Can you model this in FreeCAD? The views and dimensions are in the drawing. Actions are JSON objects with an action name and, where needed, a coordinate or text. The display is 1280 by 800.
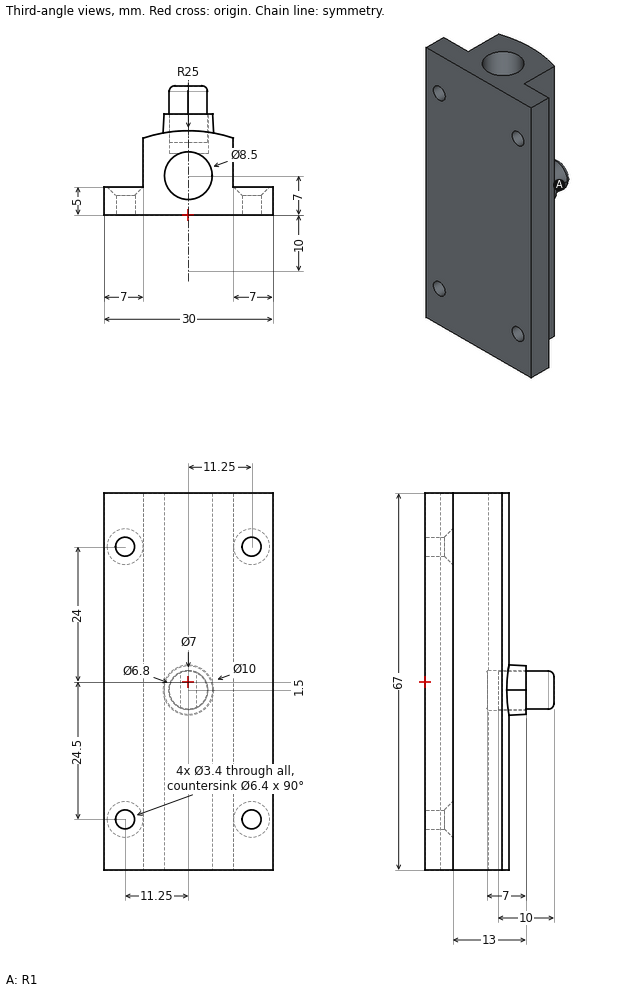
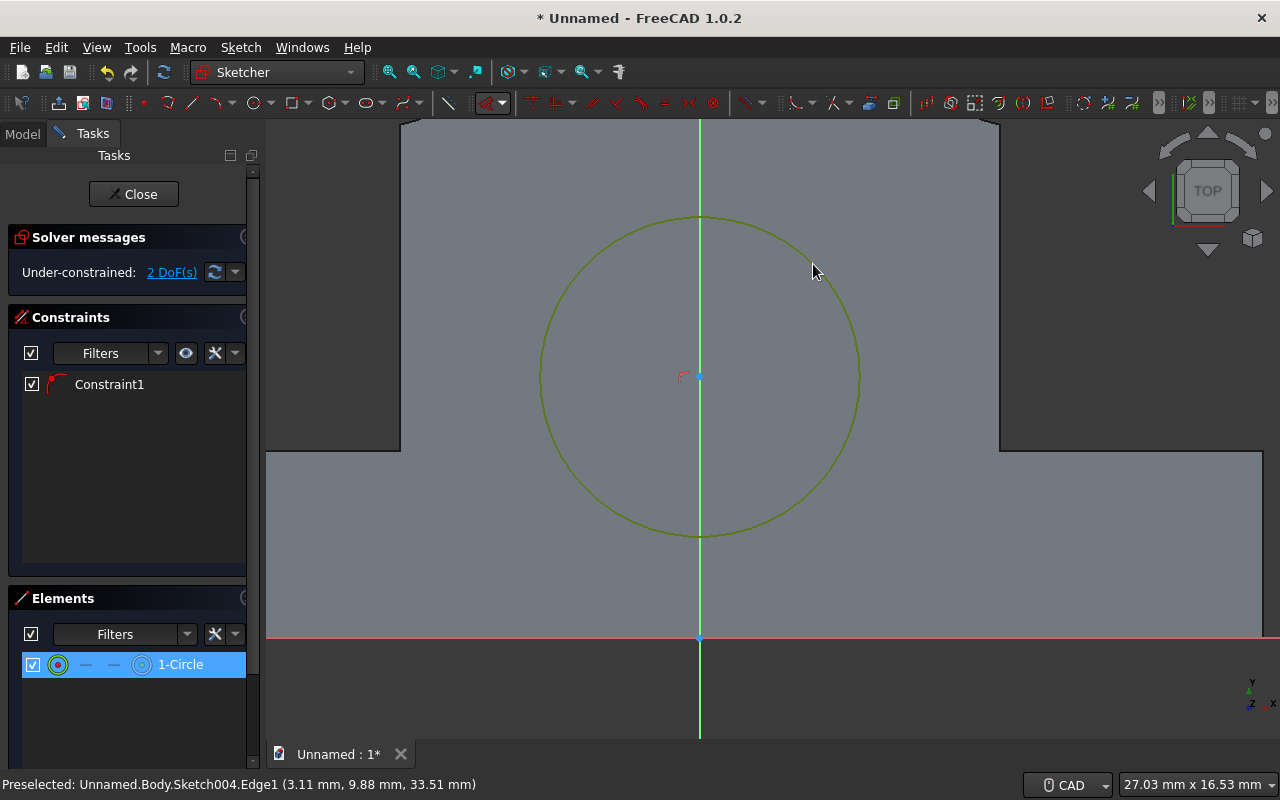
{"action": "key", "text": "k o"}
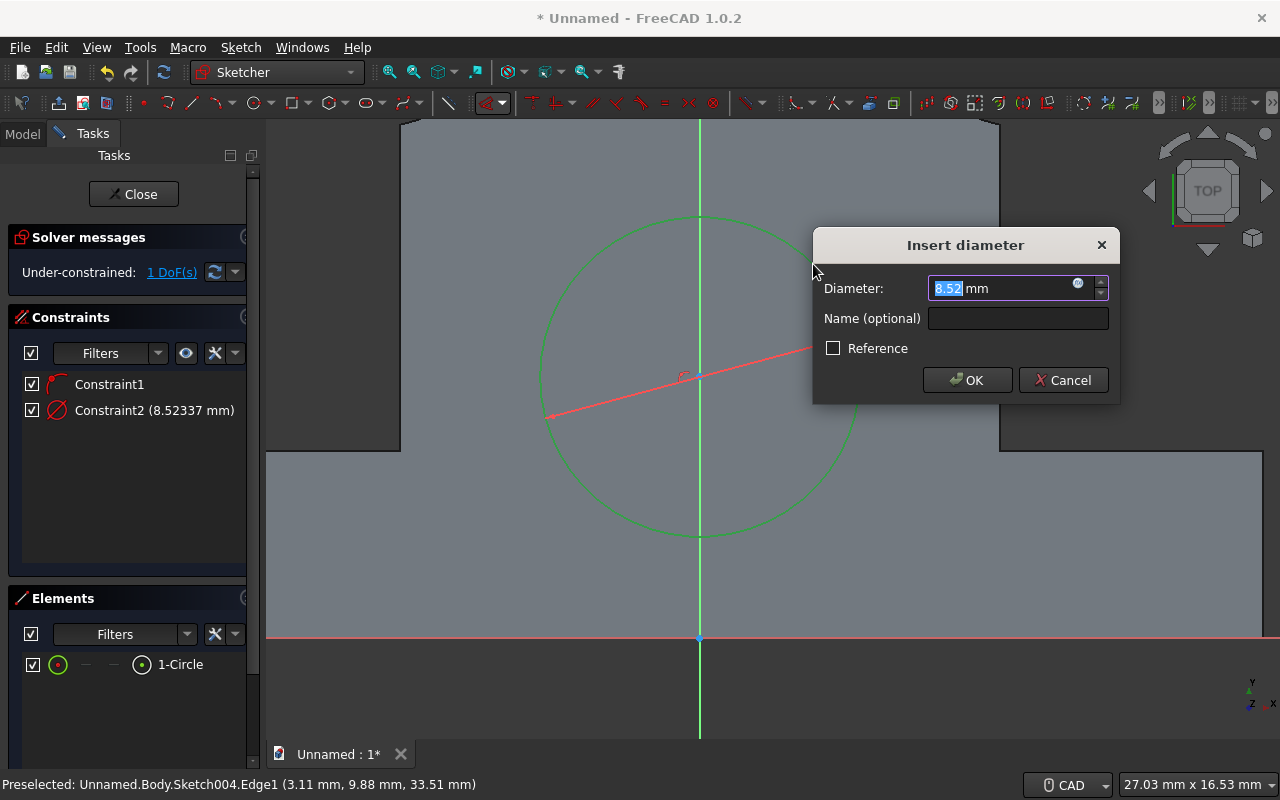
{"action": "type", "text": "8.5"}
{"action": "key", "text": "Return"}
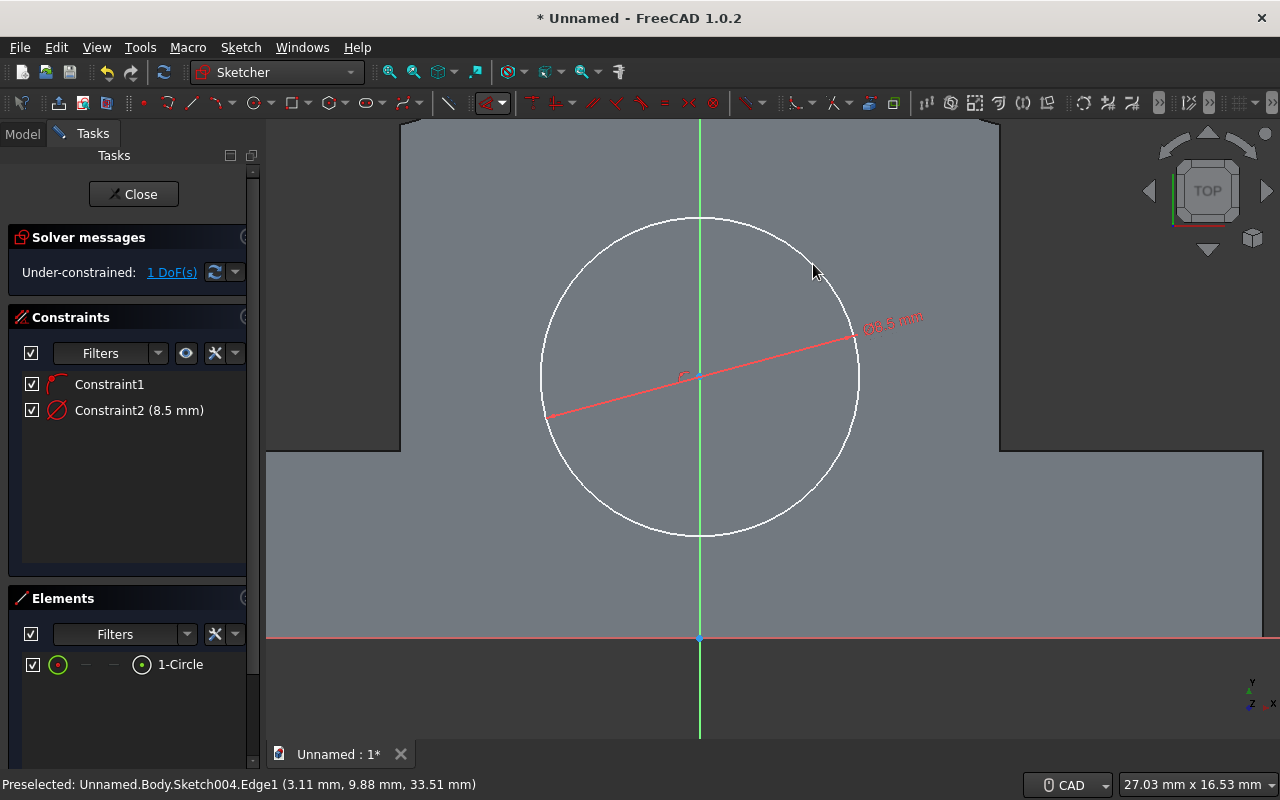
{"action": "left_click", "coordinate": [700, 377]}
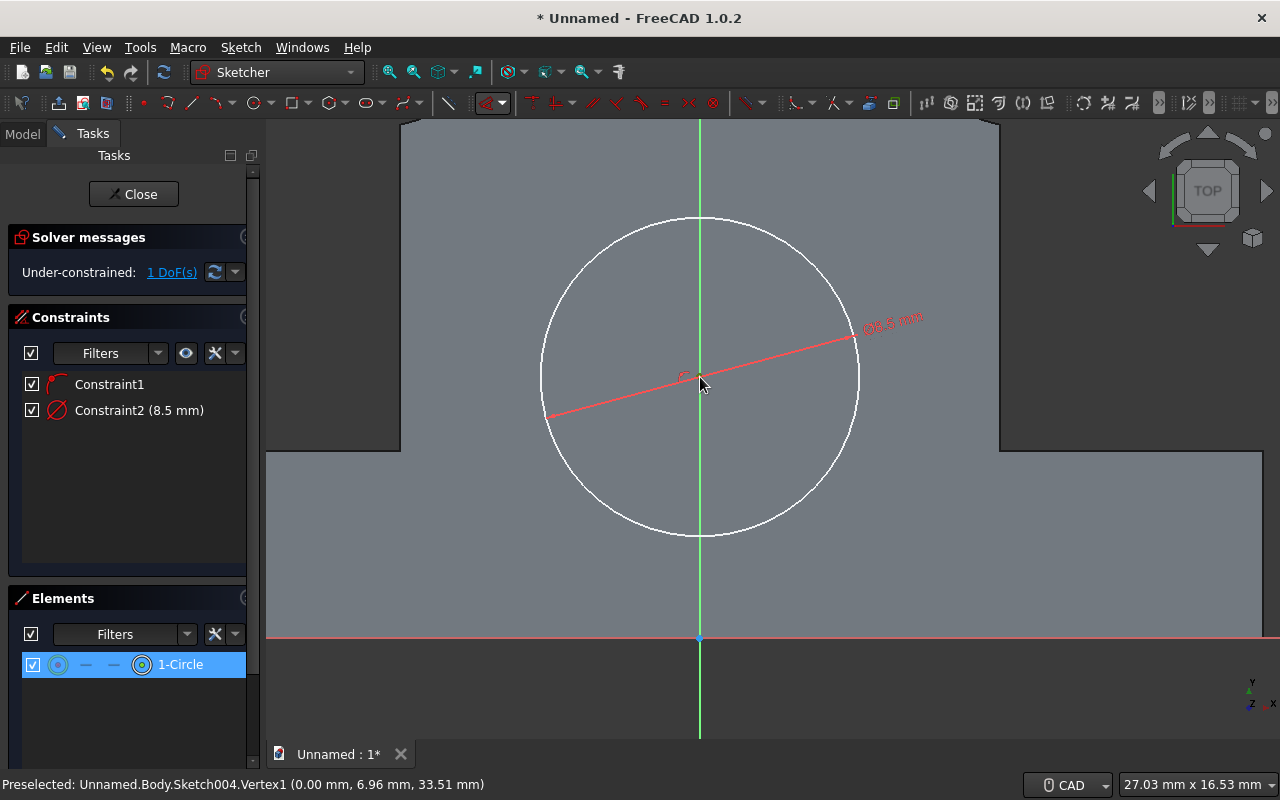
{"action": "key", "text": "i"}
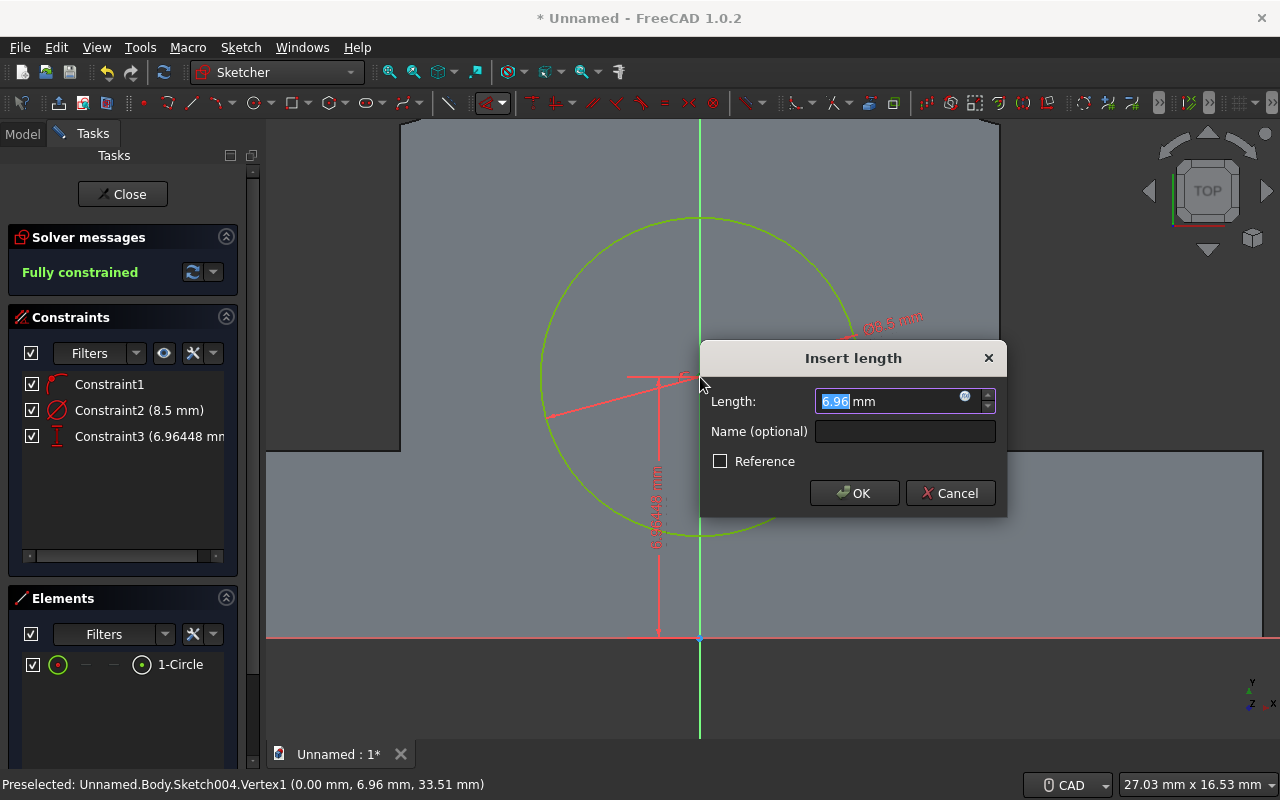
{"action": "type", "text": "7"}
{"action": "key", "text": "Return"}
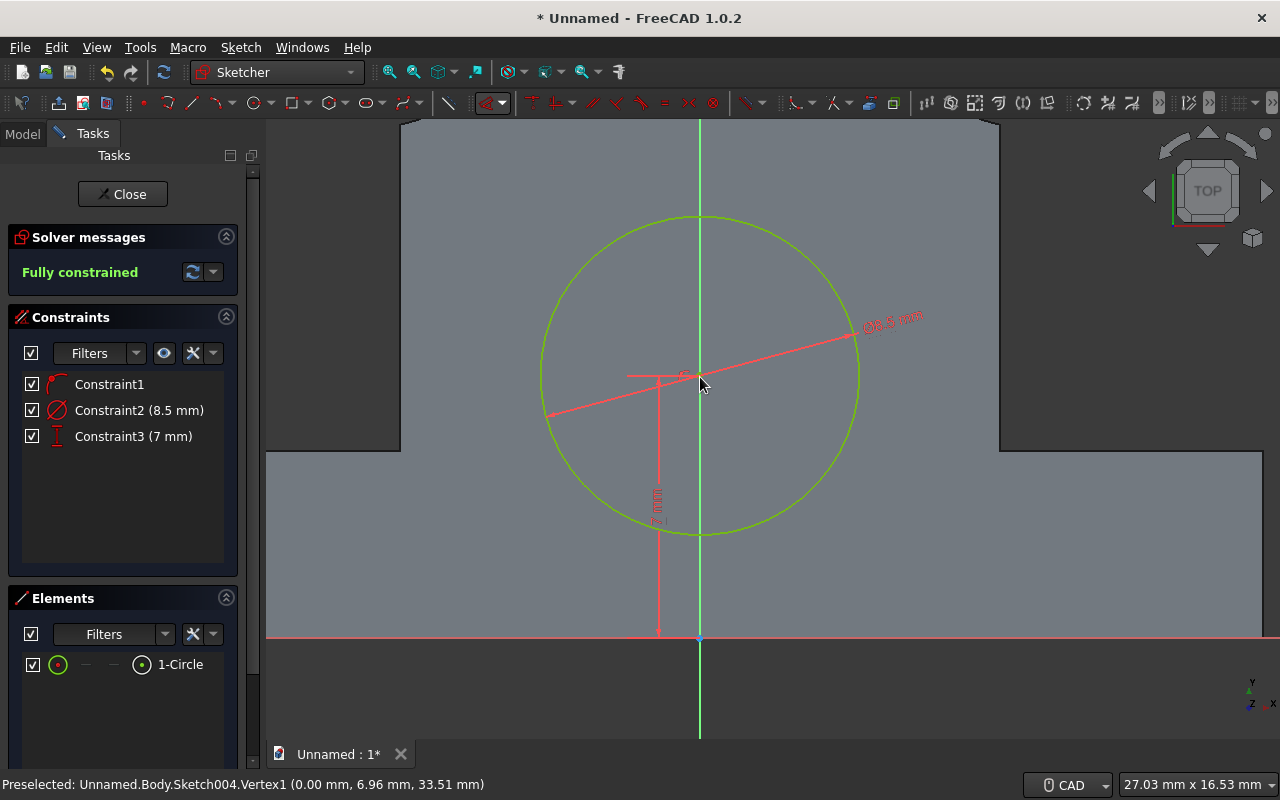
{"action": "left_click", "coordinate": [123, 194]}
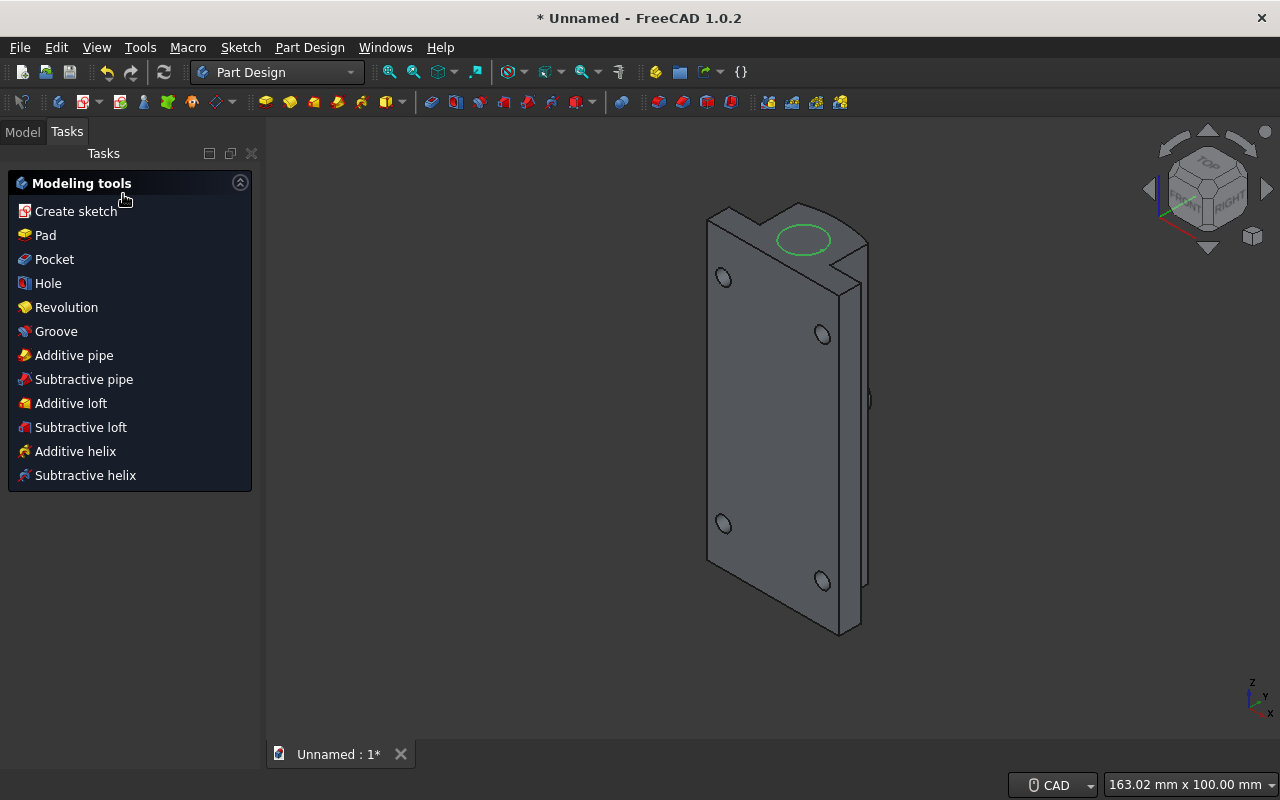
{"action": "left_click", "coordinate": [432, 102]}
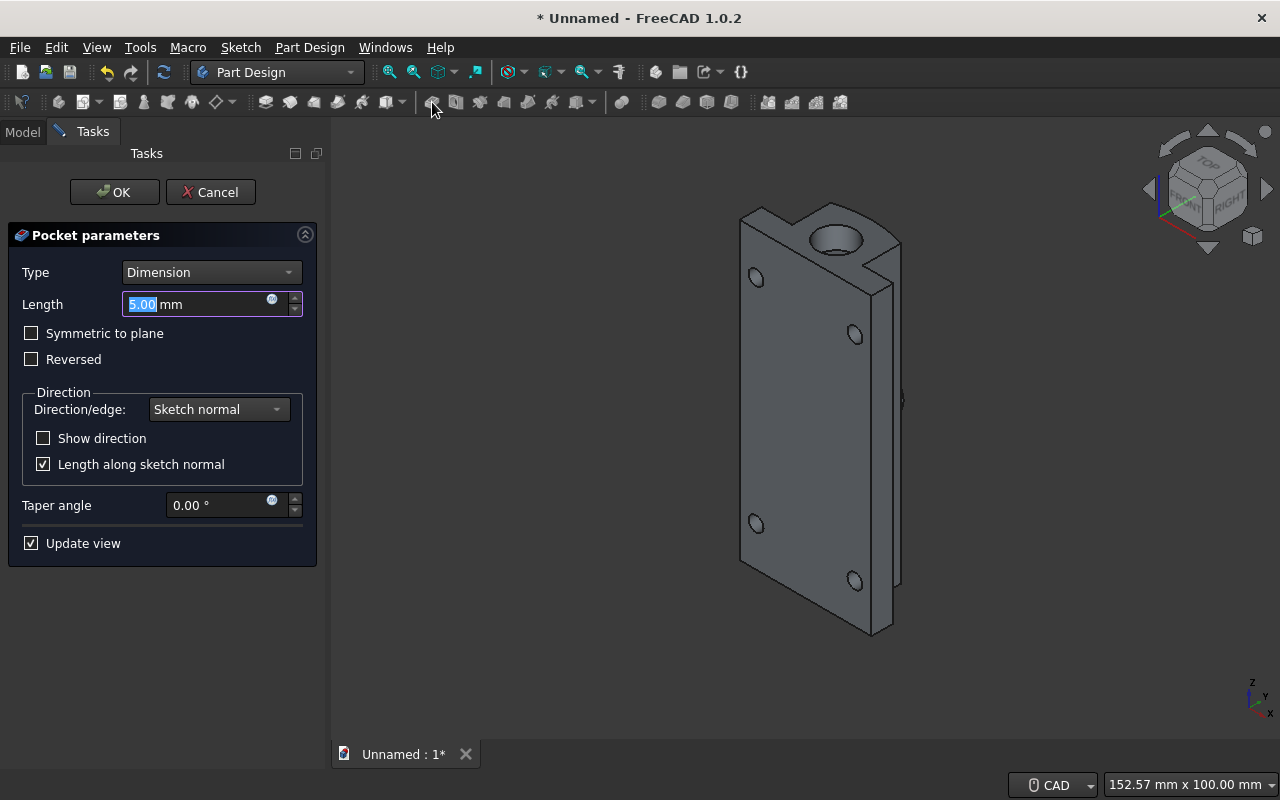
{"action": "left_click", "coordinate": [212, 272]}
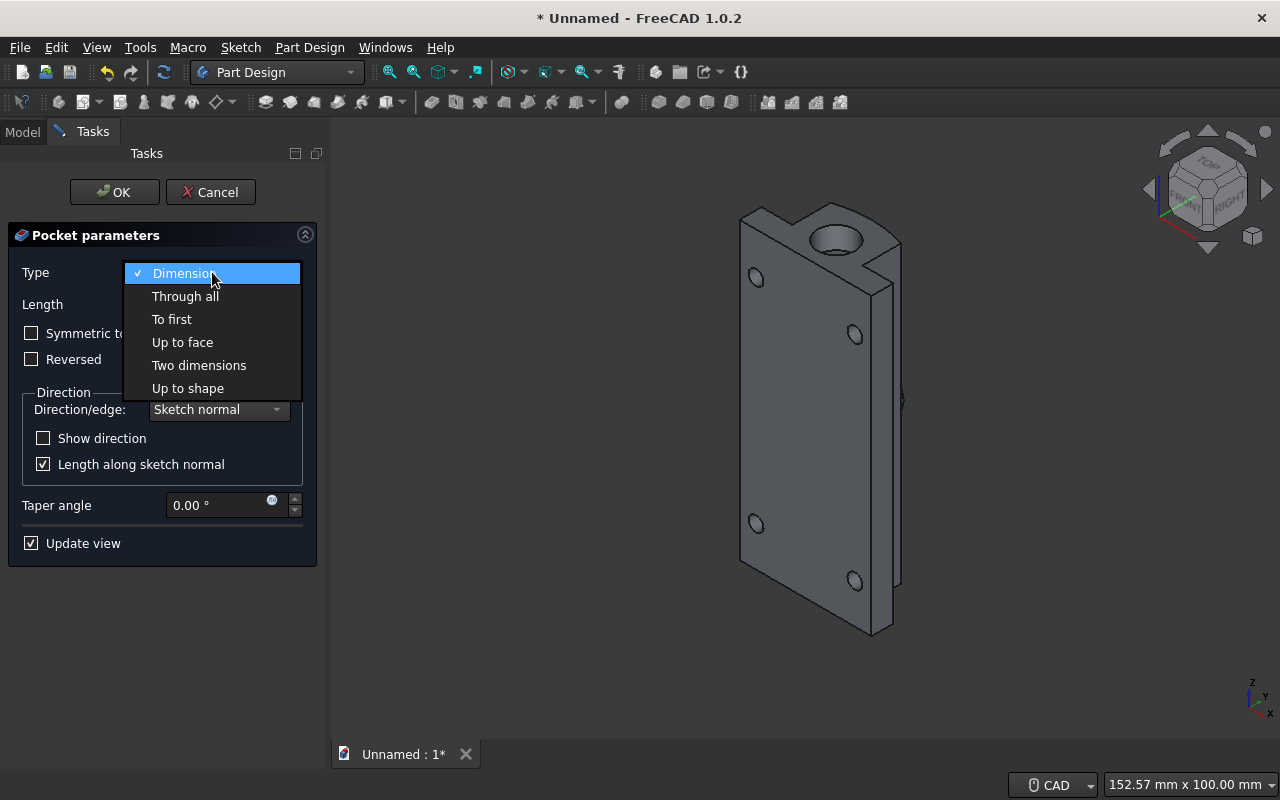
{"action": "left_click", "coordinate": [212, 296]}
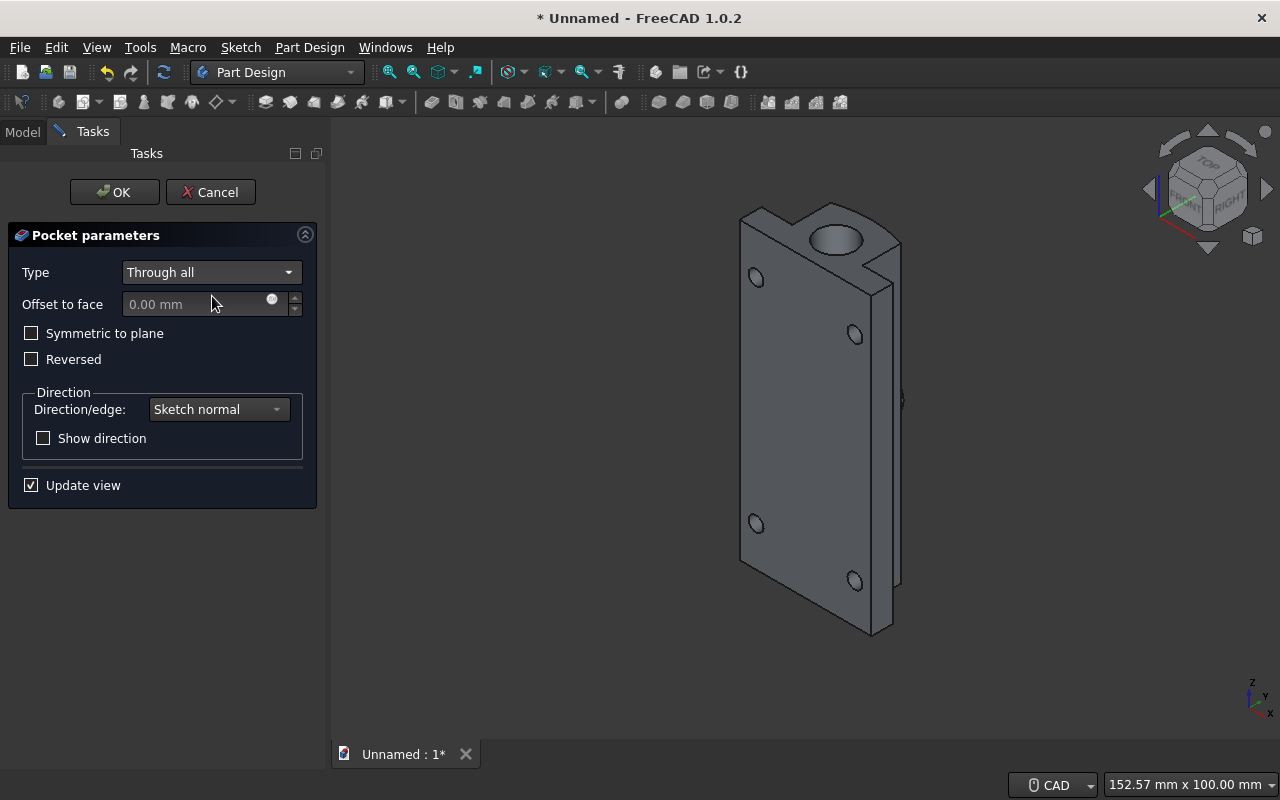
{"action": "left_click", "coordinate": [115, 192]}